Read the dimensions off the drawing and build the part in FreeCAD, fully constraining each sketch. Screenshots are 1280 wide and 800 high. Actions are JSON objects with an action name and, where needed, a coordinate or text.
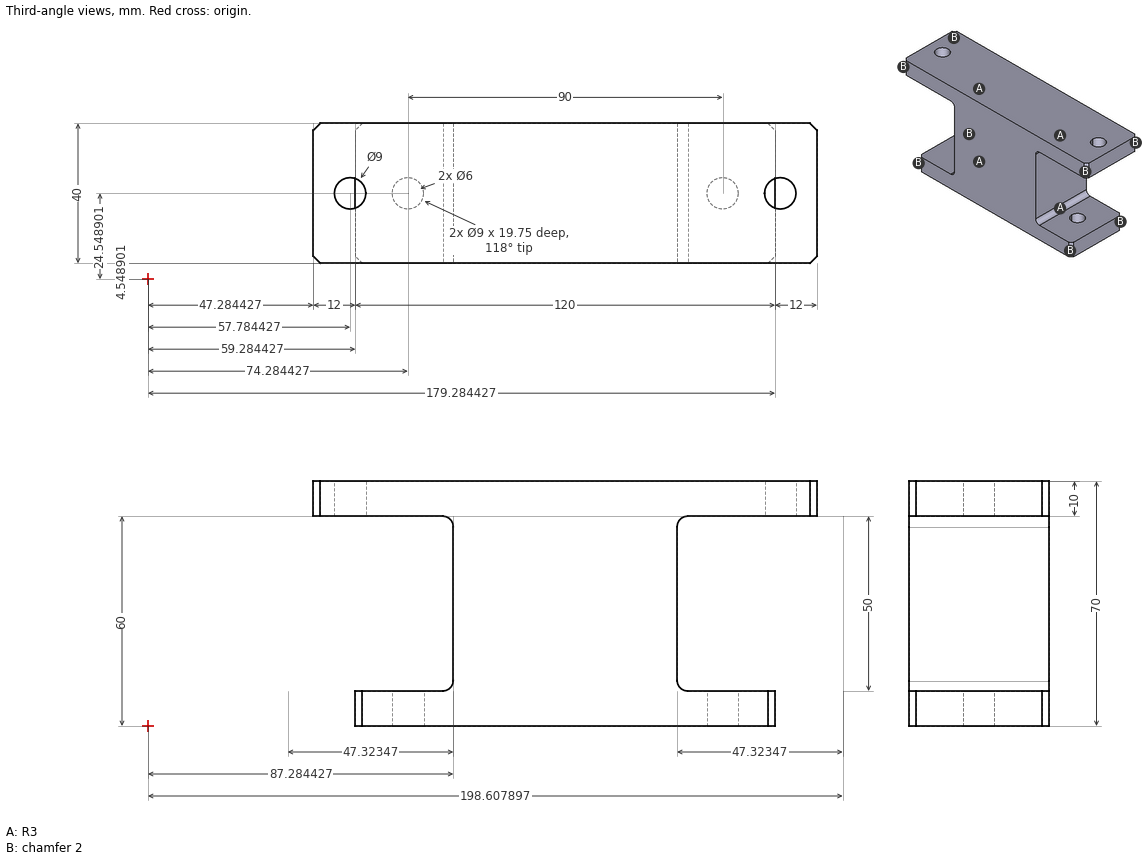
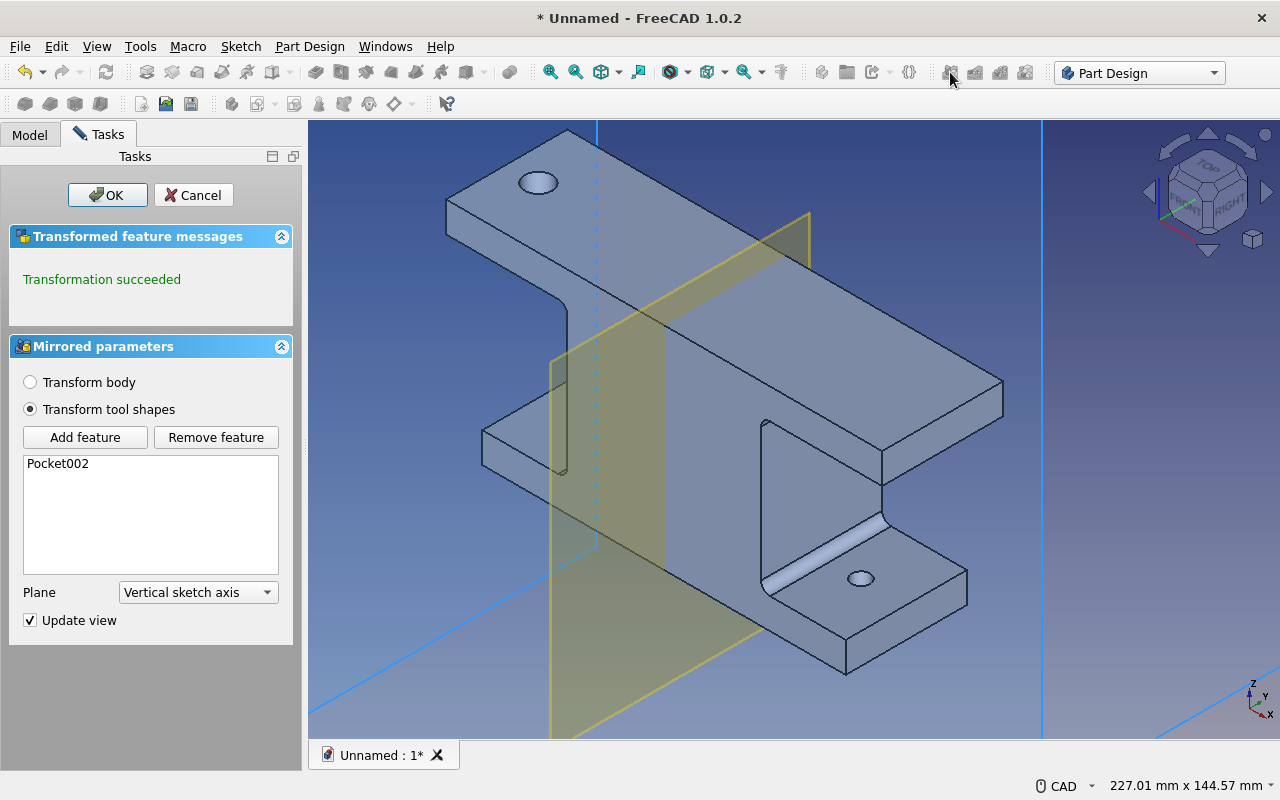
{"action": "left_click", "coordinate": [199, 592]}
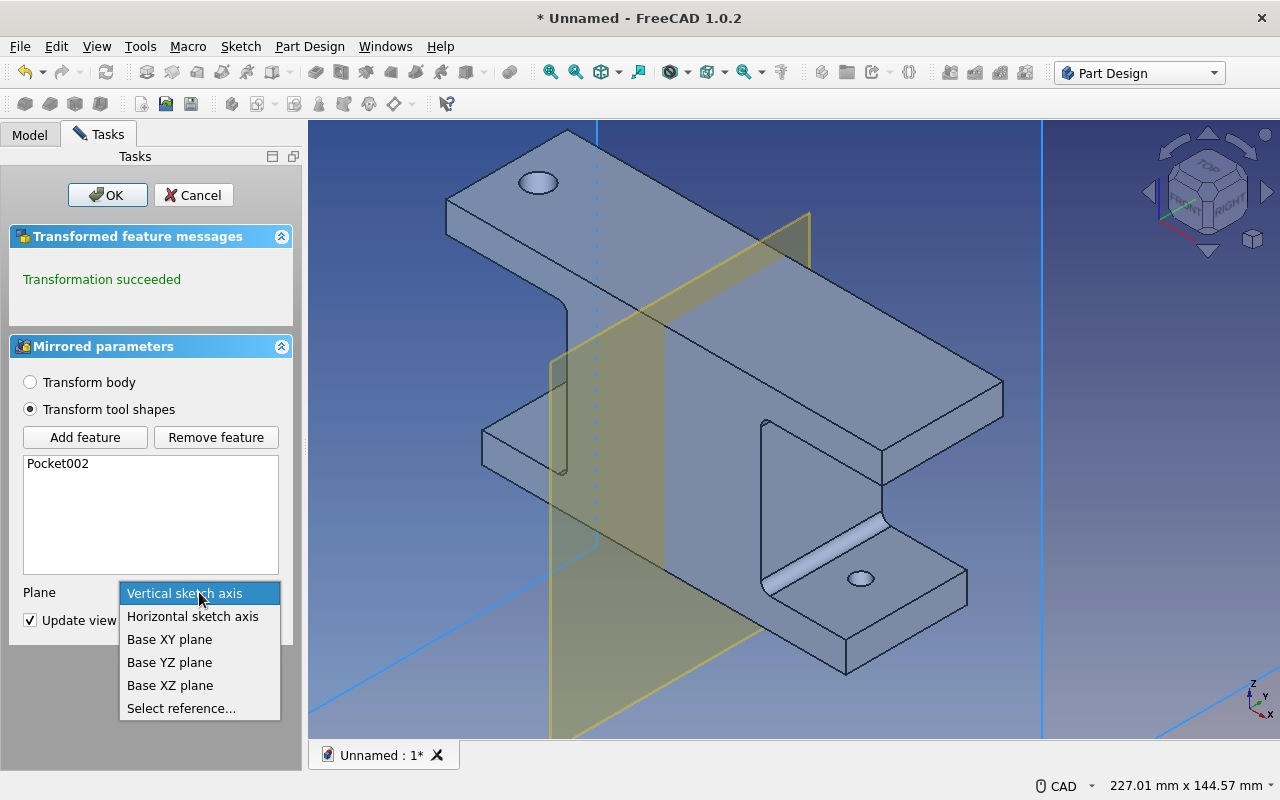
{"action": "left_click", "coordinate": [198, 708]}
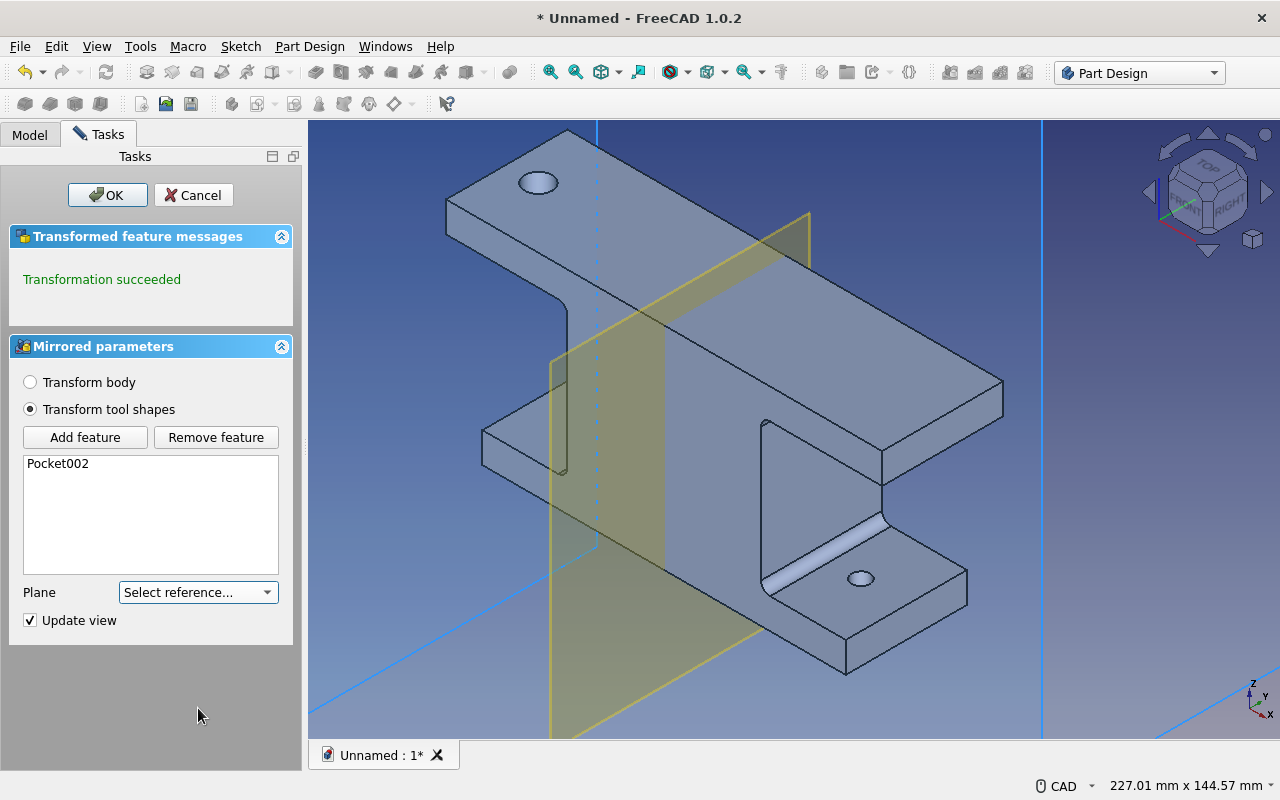
{"action": "left_click", "coordinate": [30, 134]}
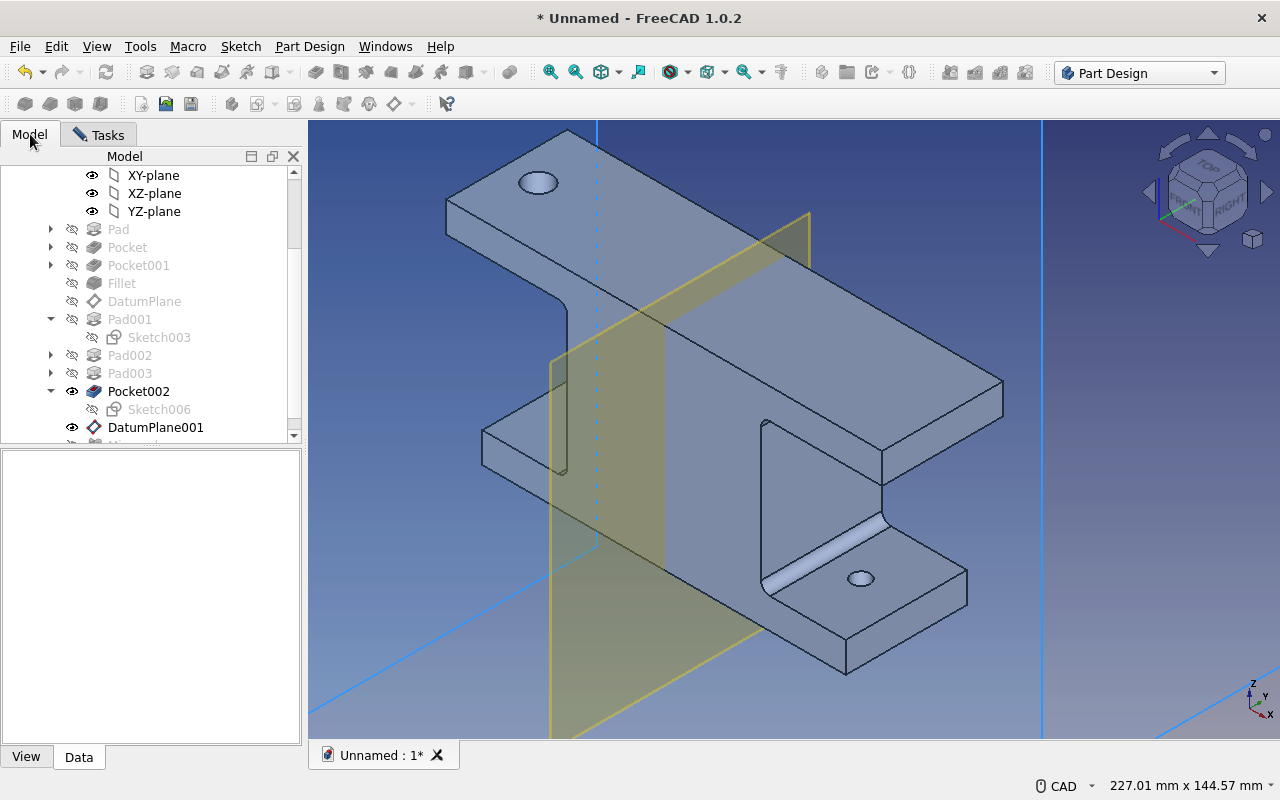
{"action": "left_click", "coordinate": [117, 427]}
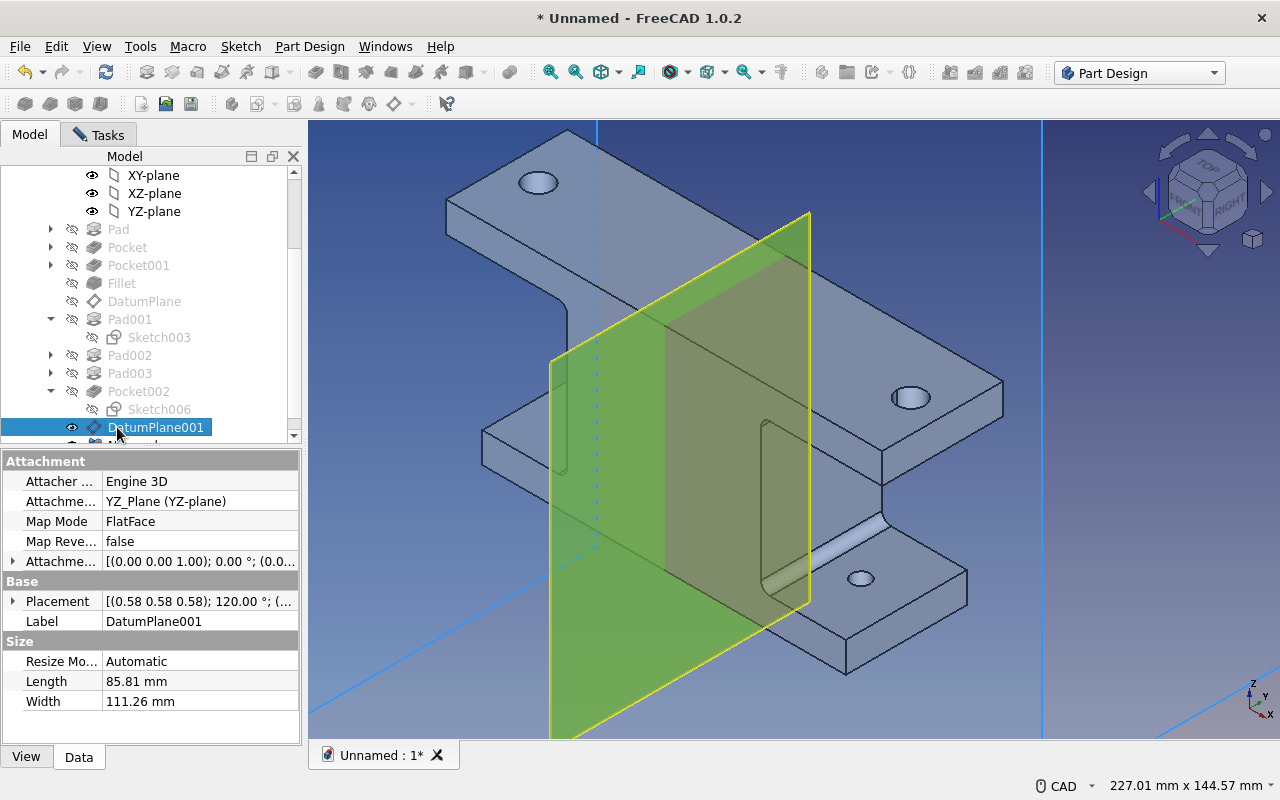
{"action": "left_click", "coordinate": [98, 134]}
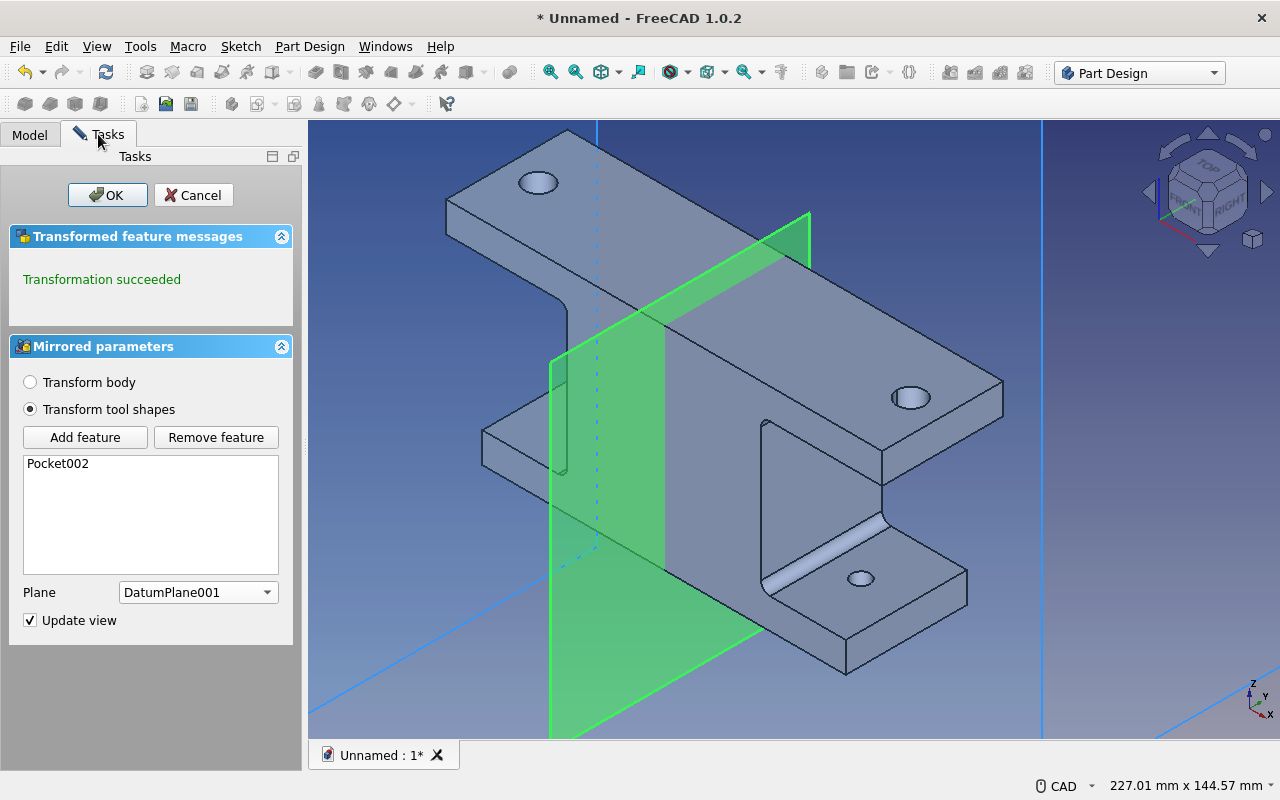
{"action": "left_click", "coordinate": [108, 195]}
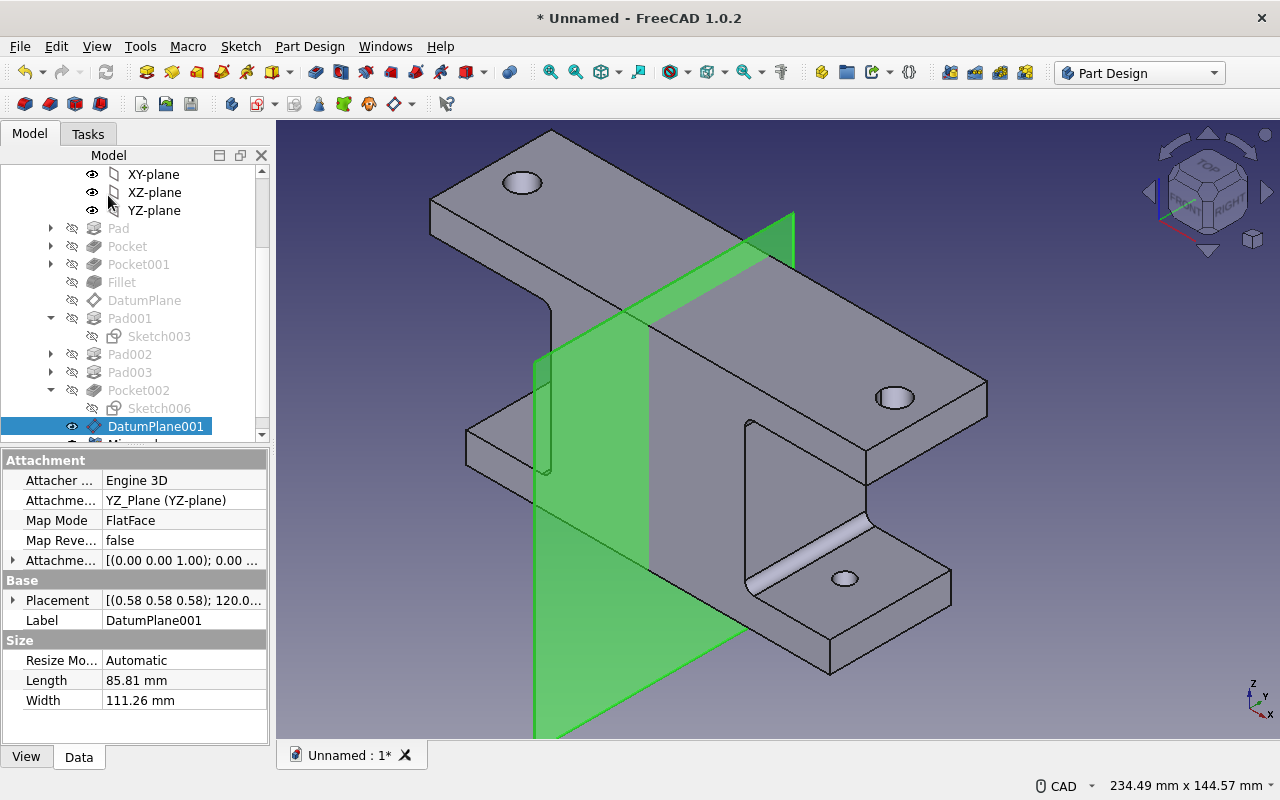
{"action": "left_click", "coordinate": [117, 426]}
{"action": "key", "text": "space"}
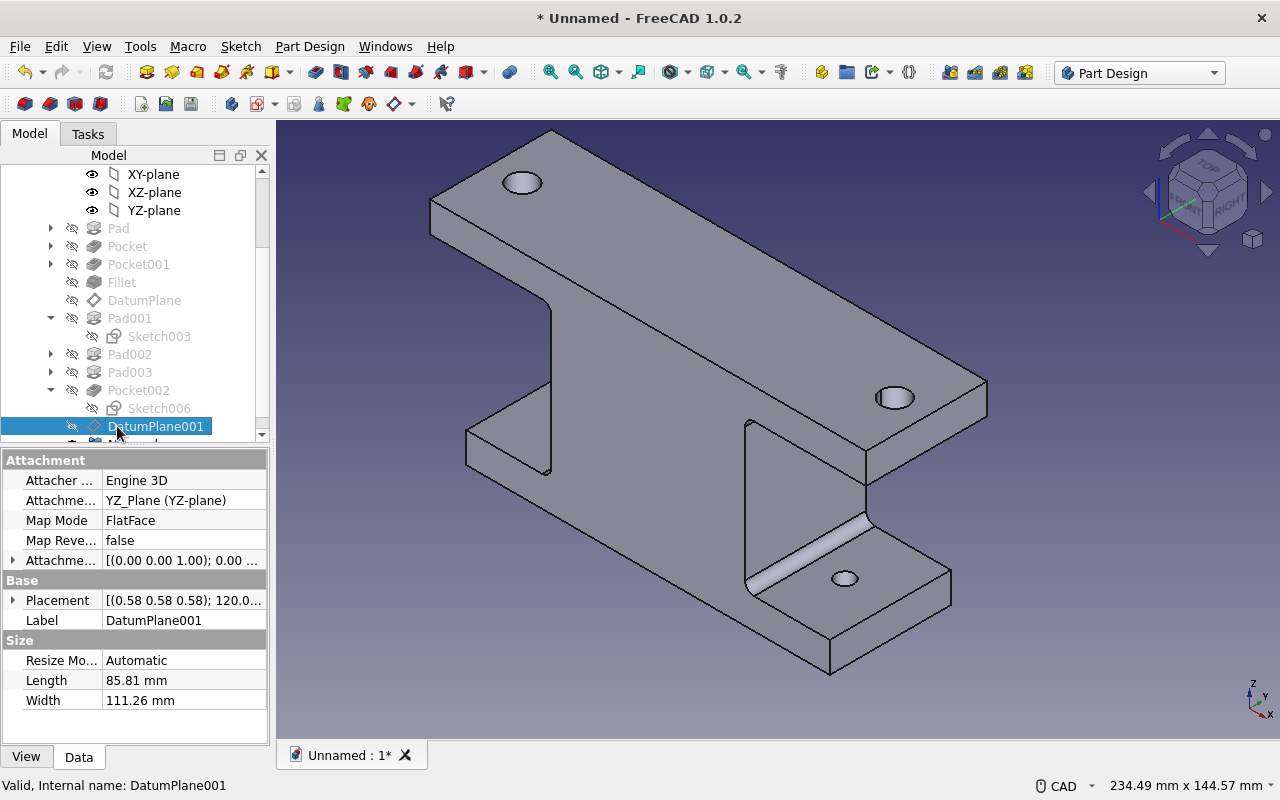
{"action": "left_click", "coordinate": [830, 656]}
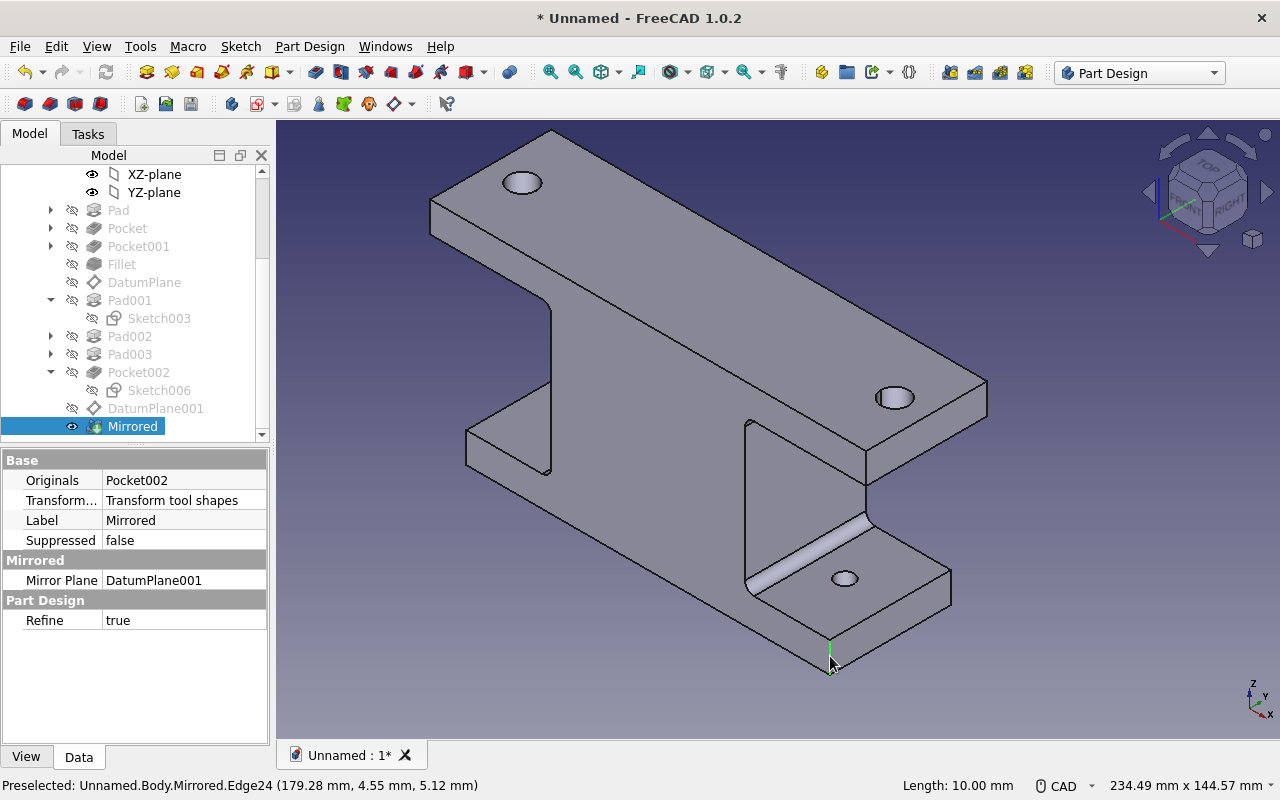
{"action": "left_click", "coordinate": [866, 468], "text": "ctrl"}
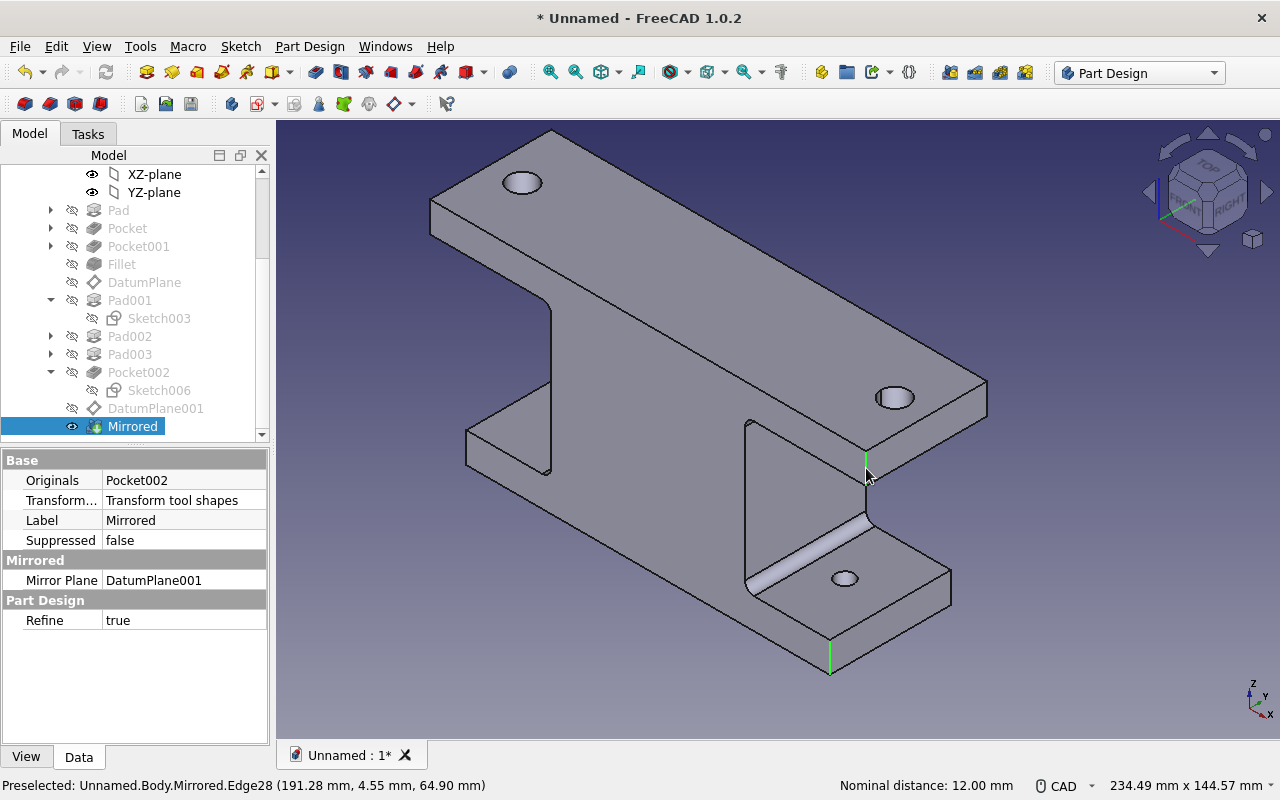
{"action": "key", "text": "2"}